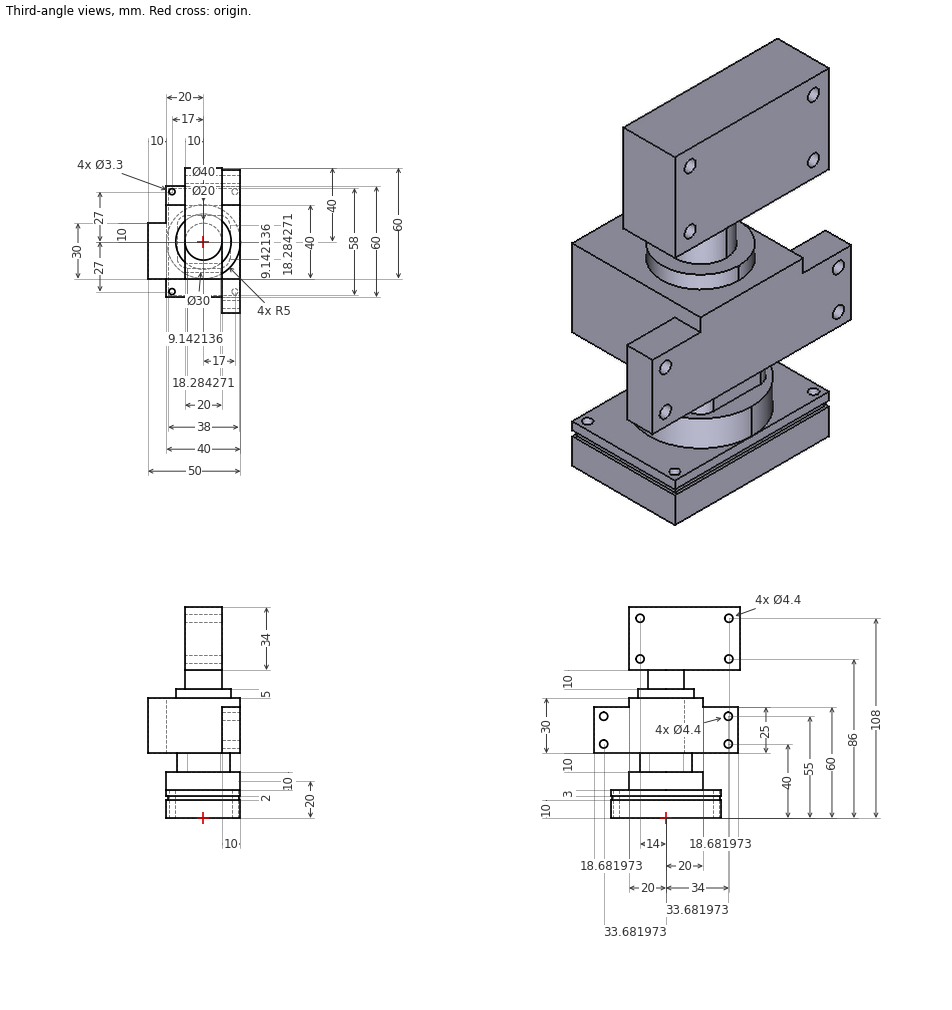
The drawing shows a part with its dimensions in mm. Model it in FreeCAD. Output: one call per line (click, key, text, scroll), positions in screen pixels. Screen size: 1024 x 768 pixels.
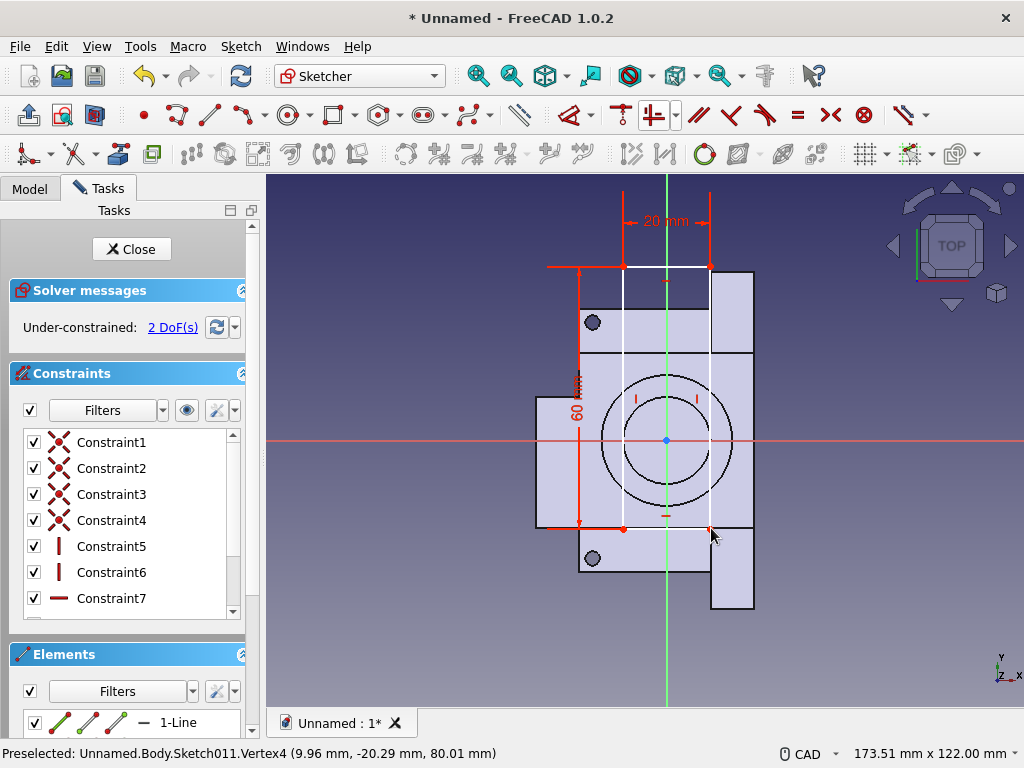
key(d)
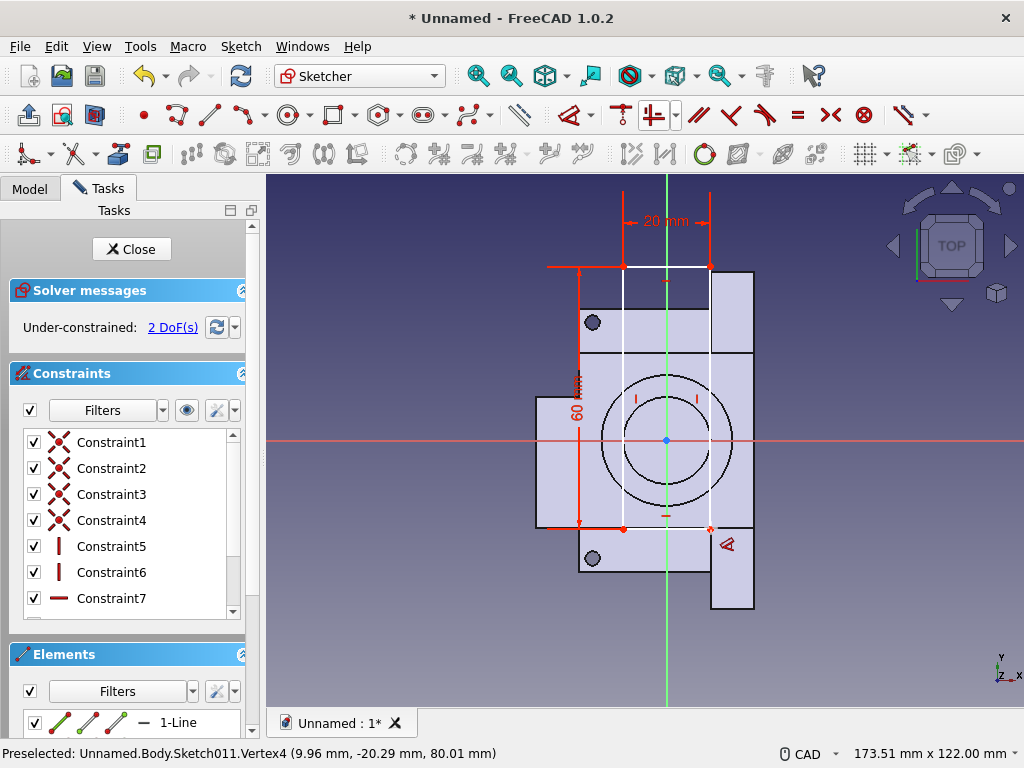
click(623, 267)
click(645, 233)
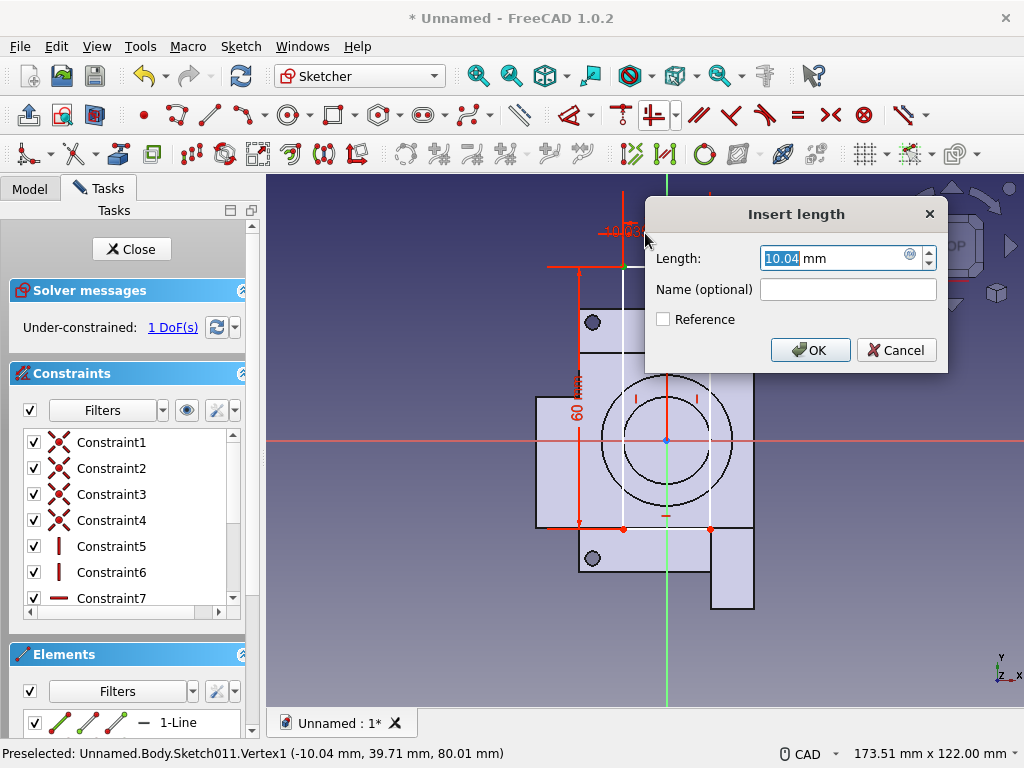
text(10)
key(Return)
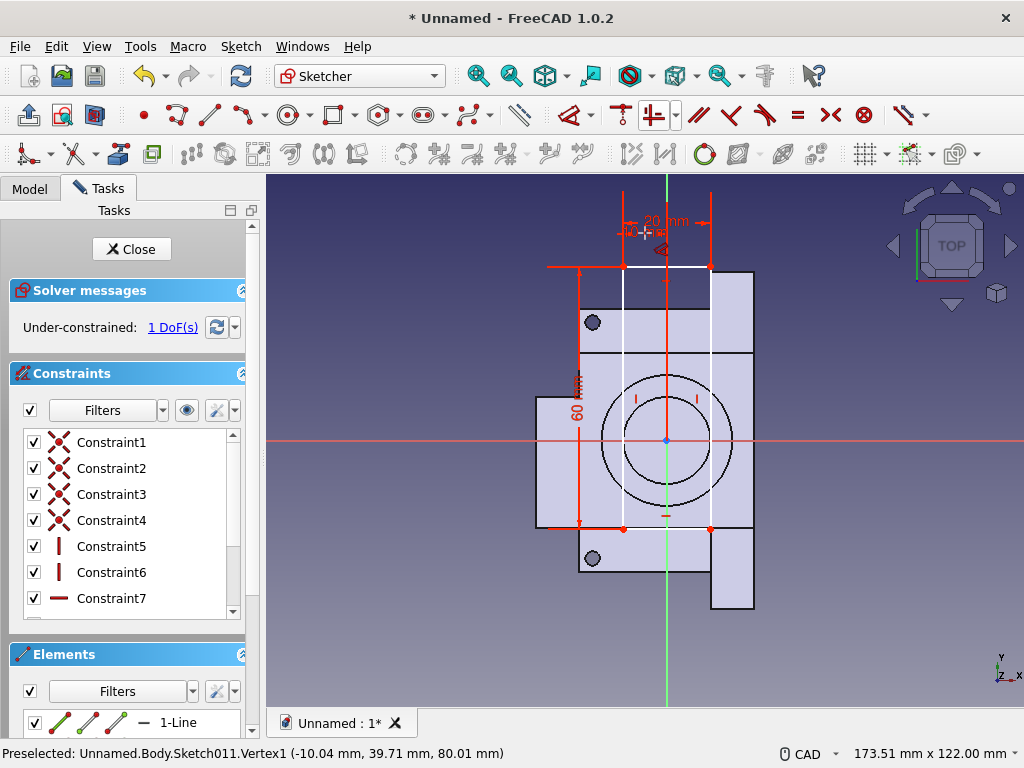
click(623, 267)
click(589, 354)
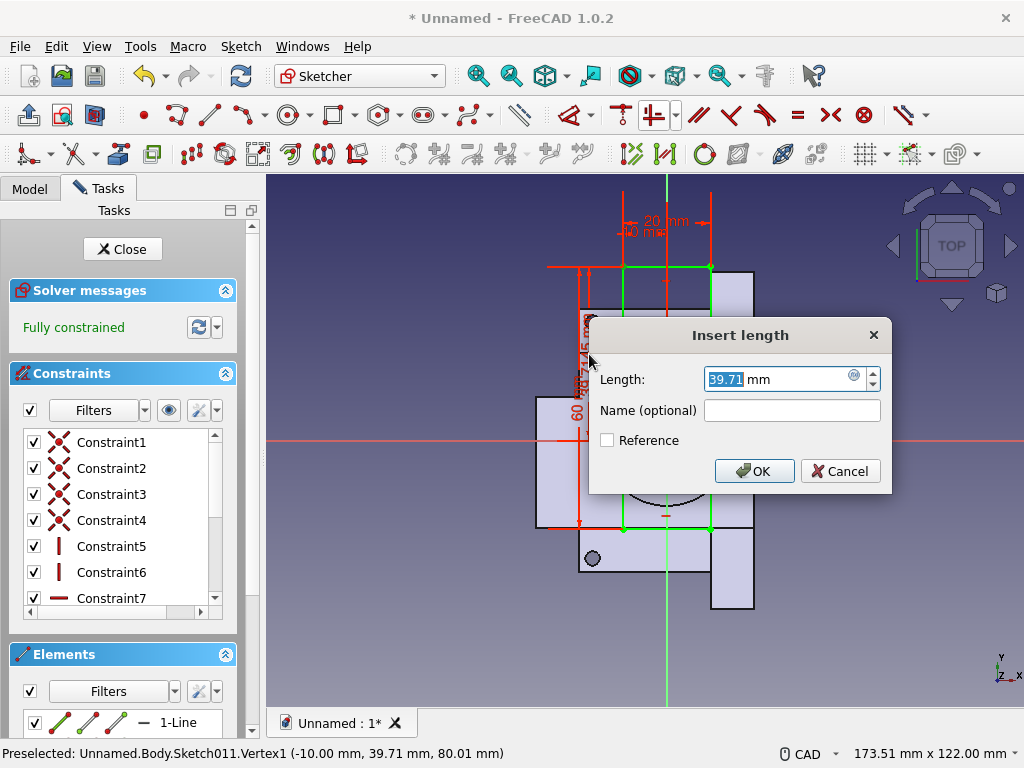
text(40)
key(Return)
key(Escape)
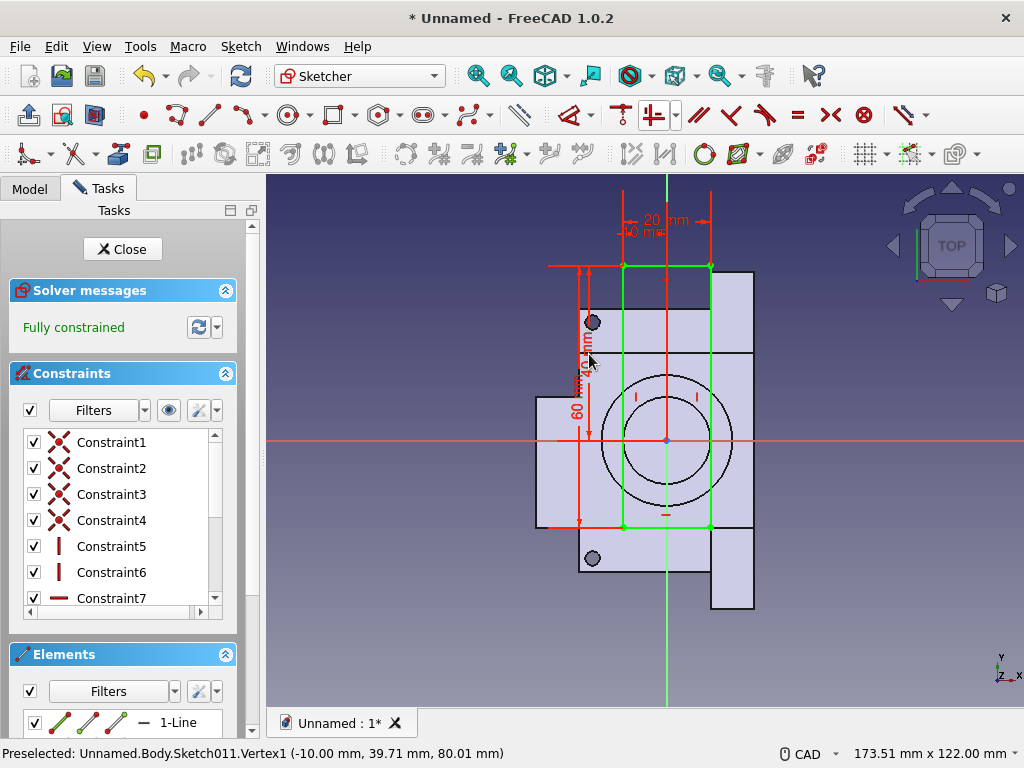
click(123, 249)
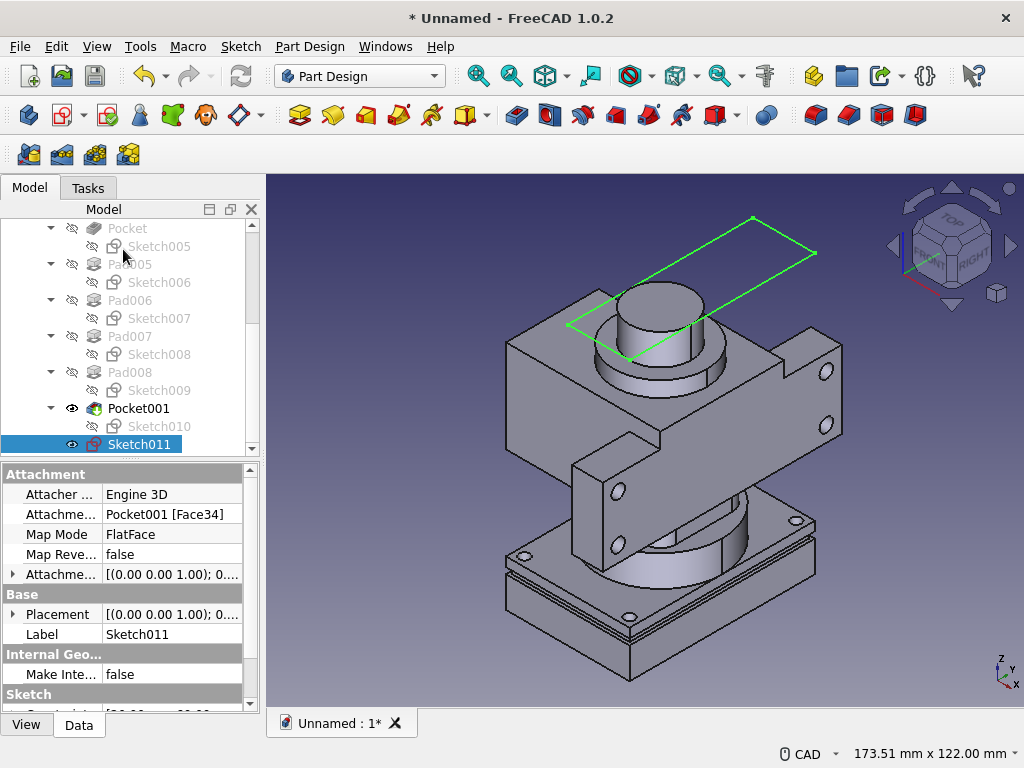
click(300, 116)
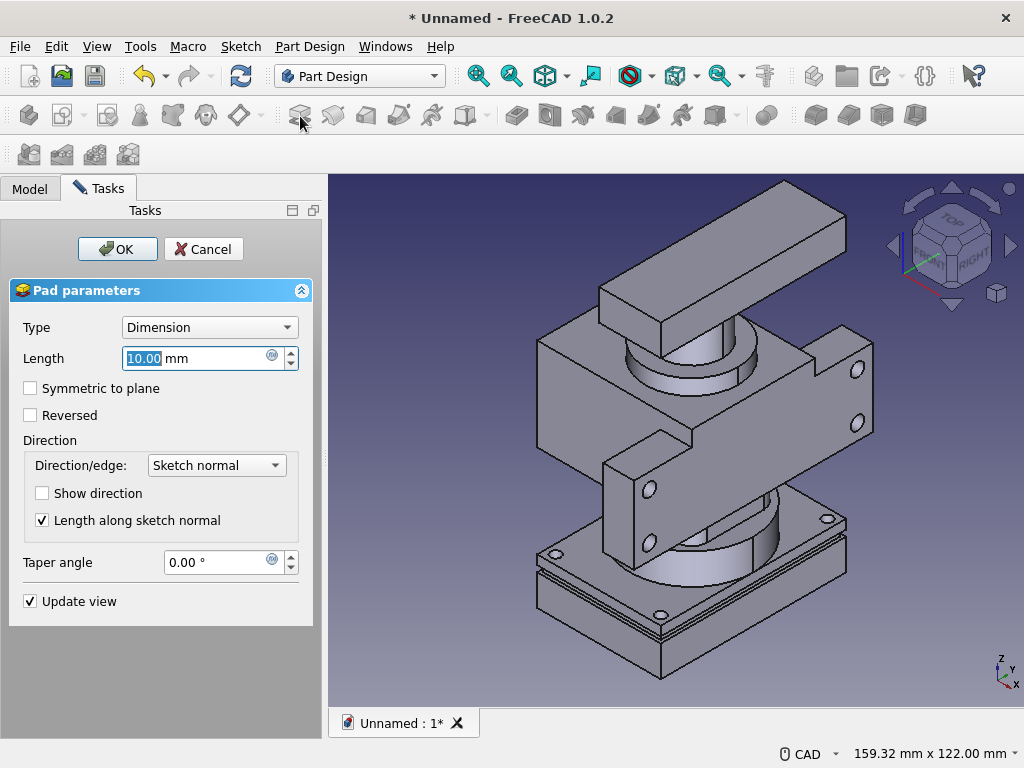
text(34)
key(Tab)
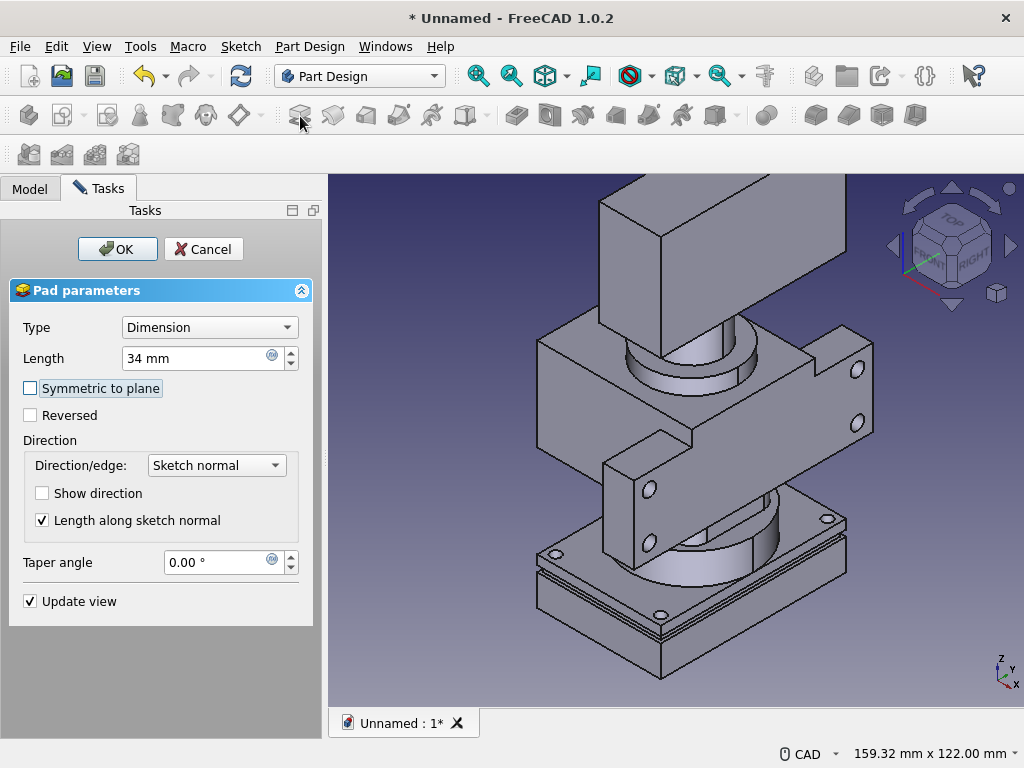
click(118, 249)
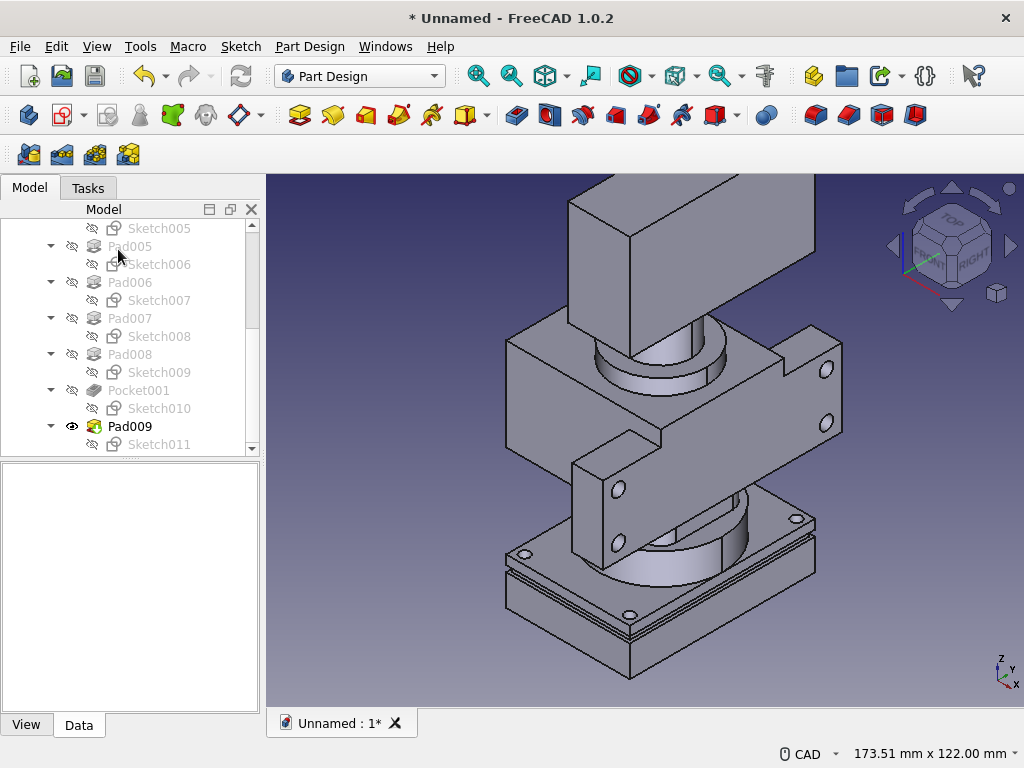
key(v)
key(f)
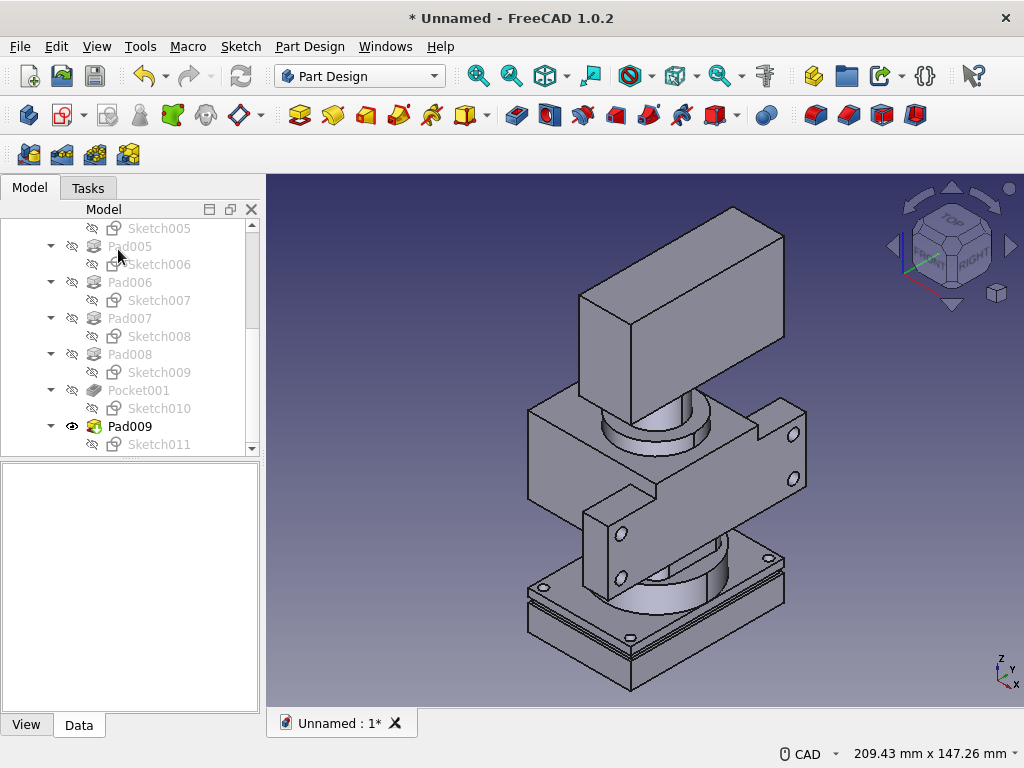
key(6)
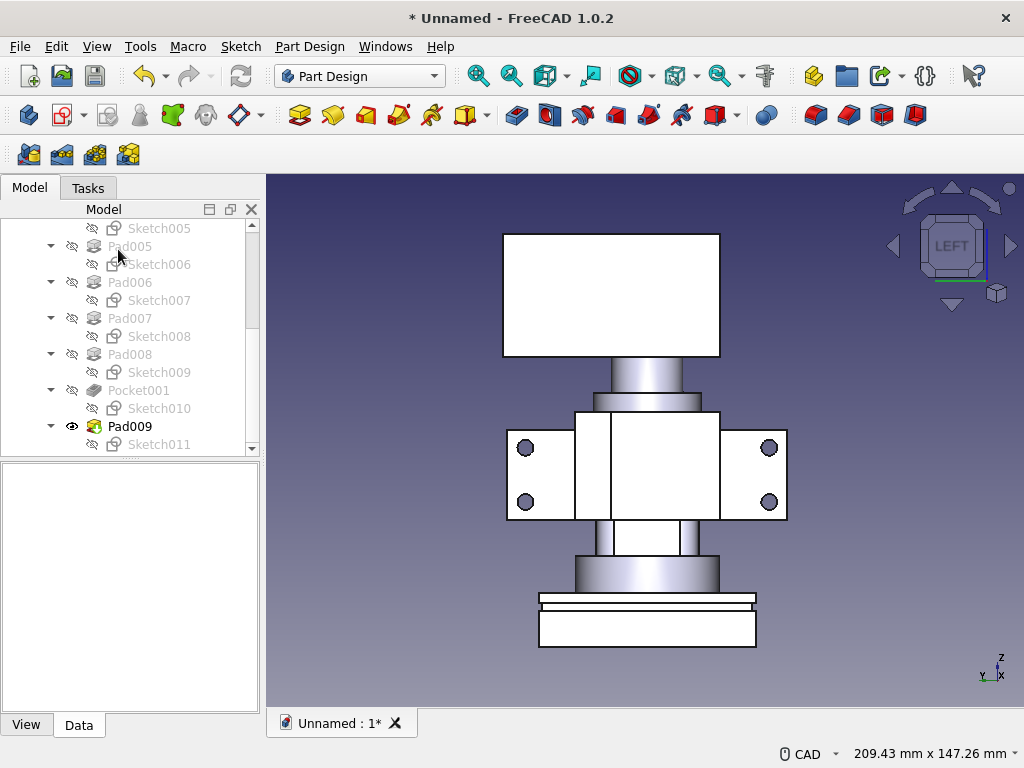
click(580, 295)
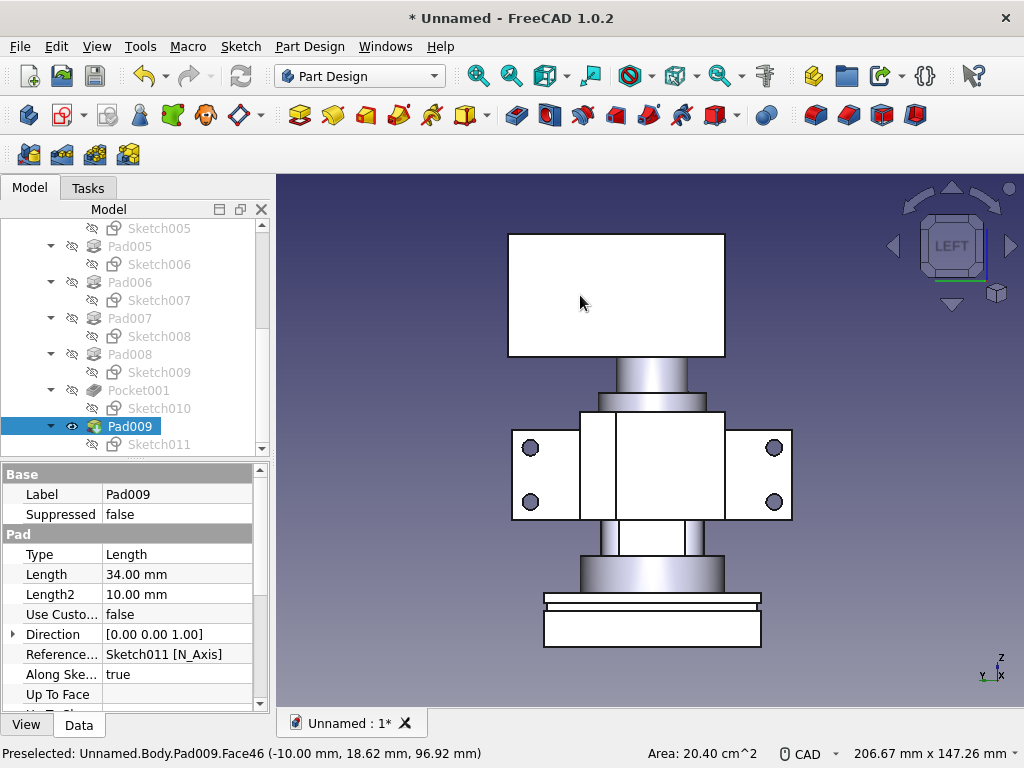
click(62, 116)